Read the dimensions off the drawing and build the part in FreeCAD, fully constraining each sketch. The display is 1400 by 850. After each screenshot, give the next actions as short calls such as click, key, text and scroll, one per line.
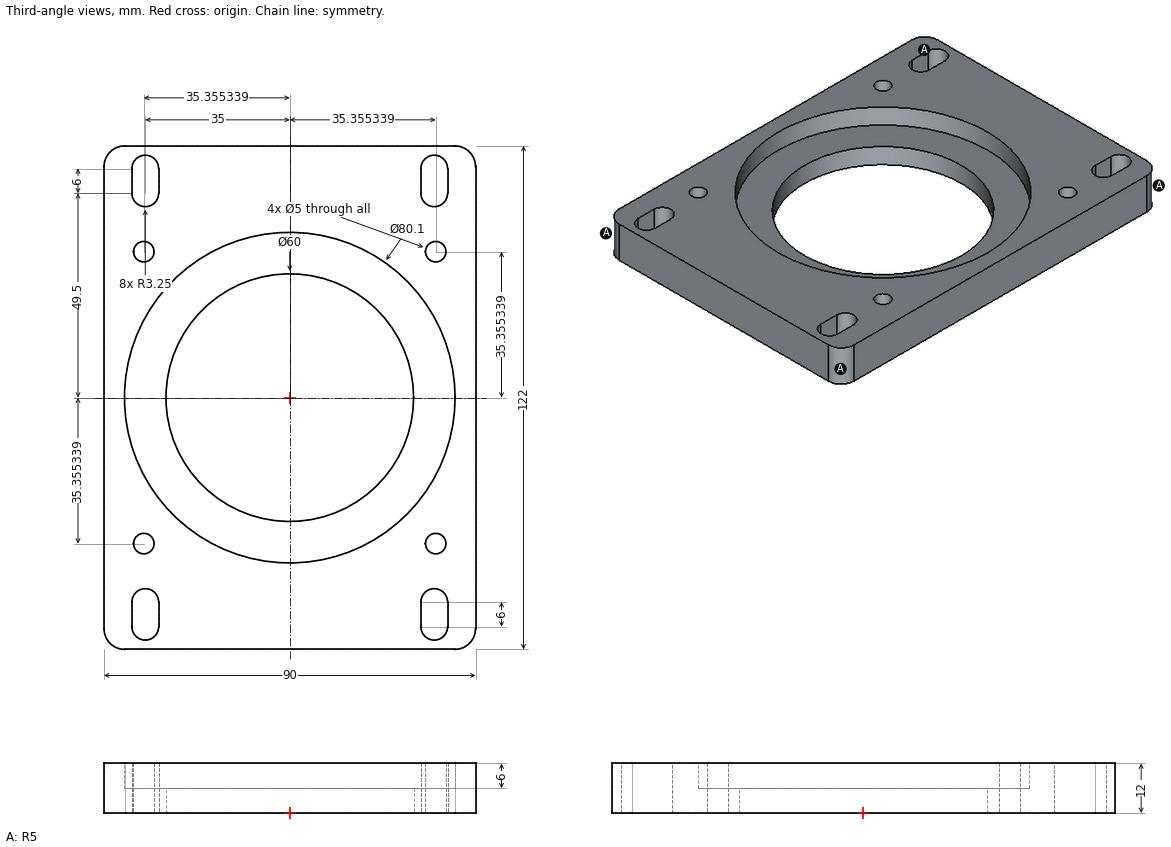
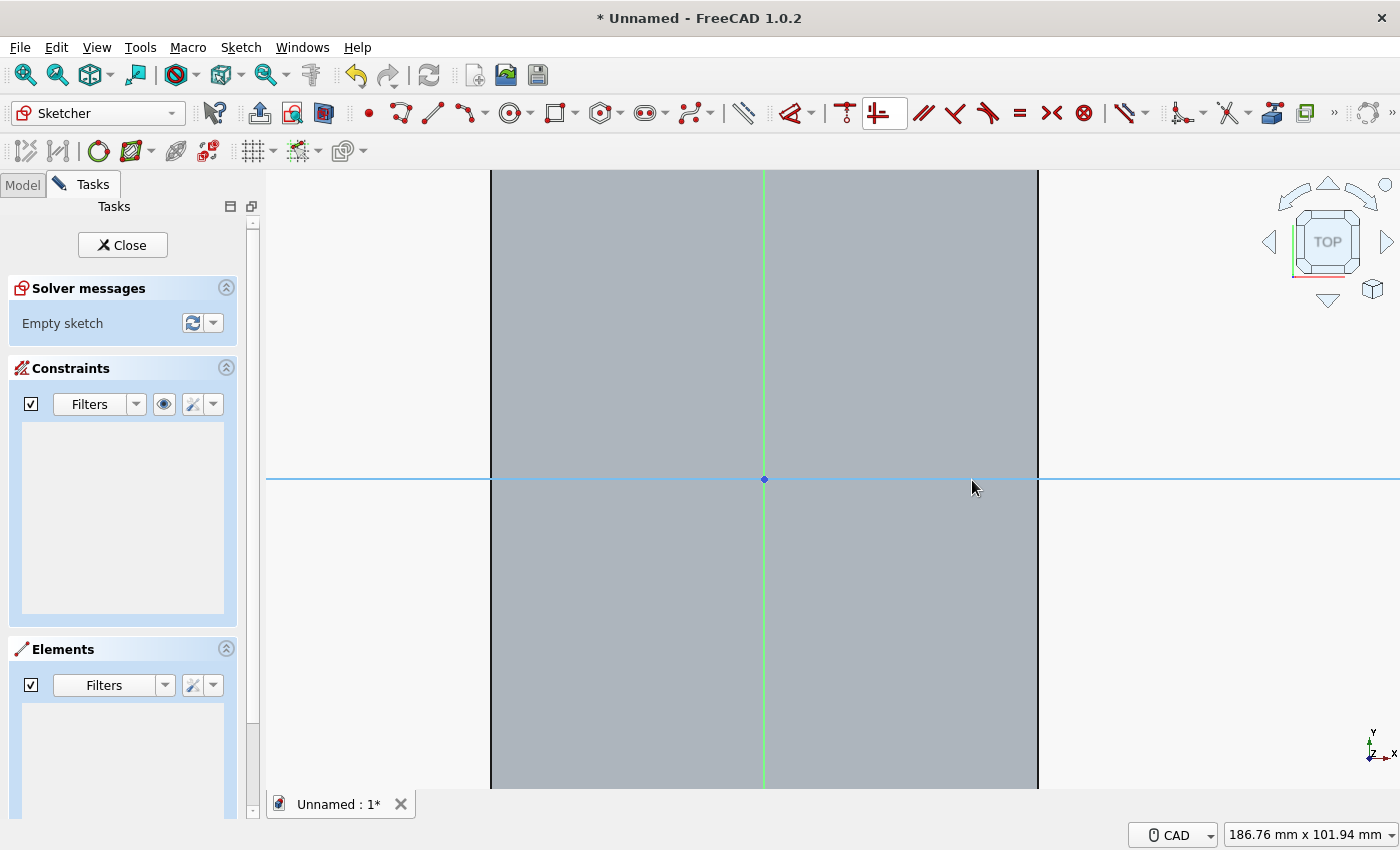
click(510, 114)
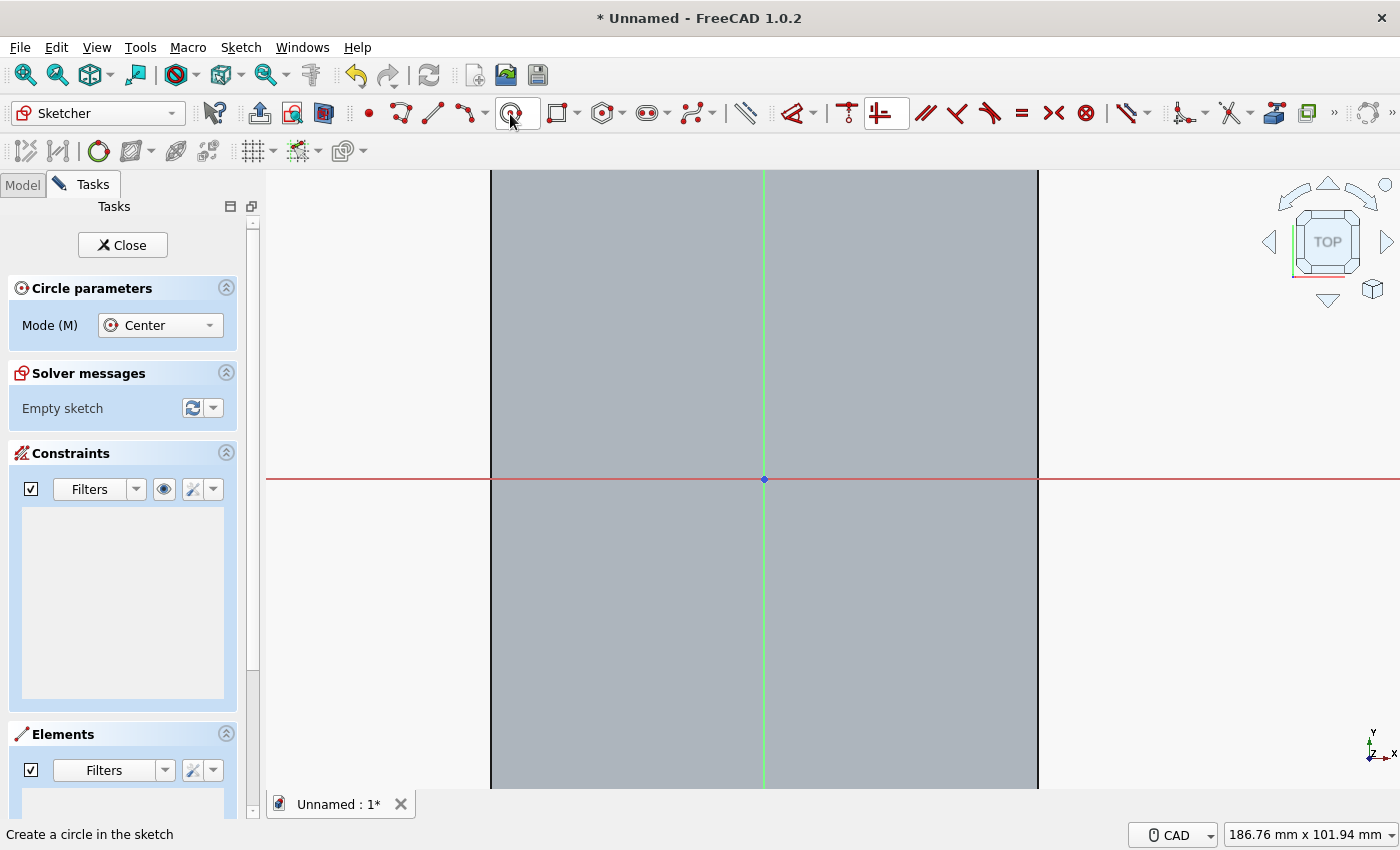
click(764, 479)
move(893, 350)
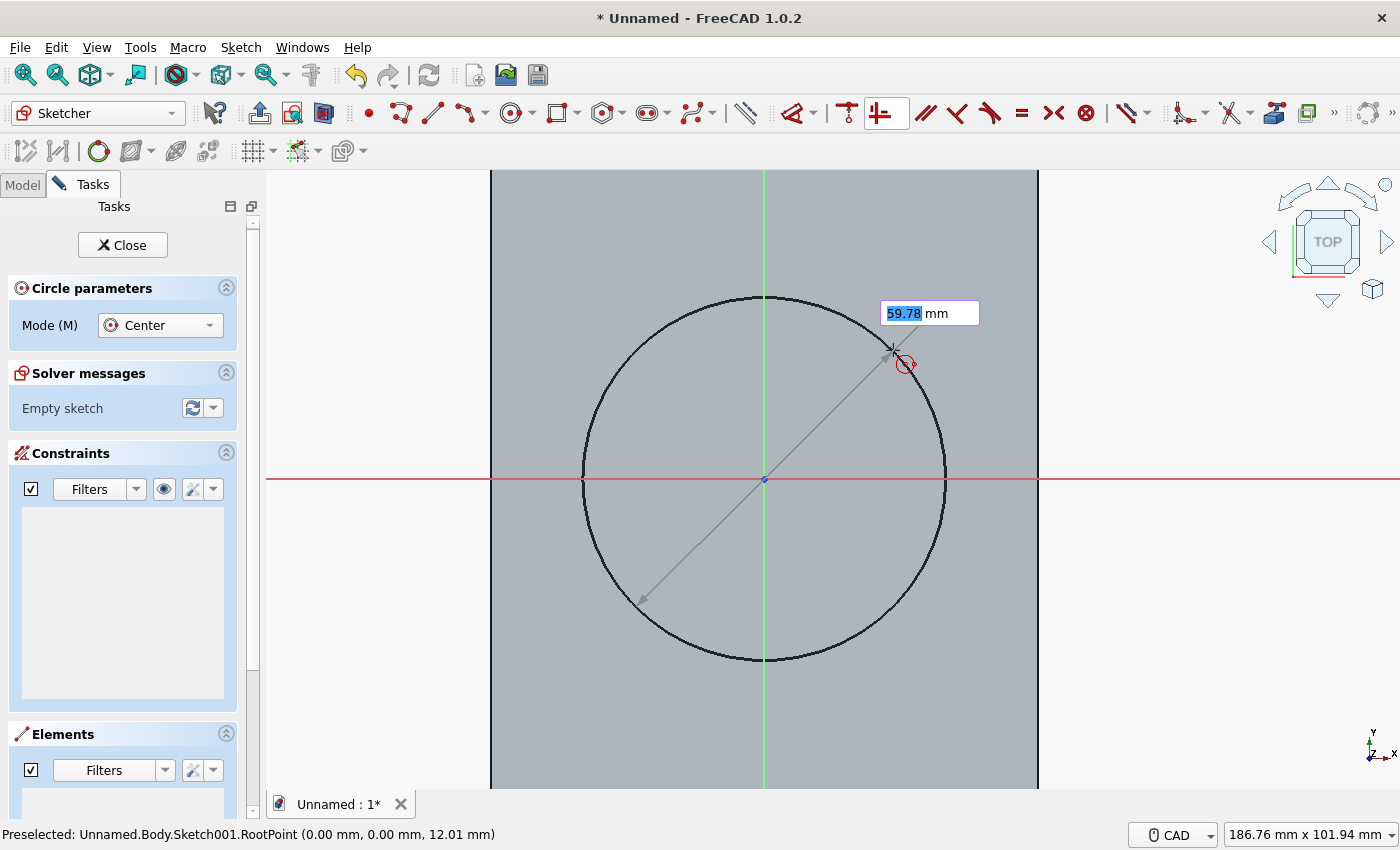
text(60)
key(Return)
key(Escape)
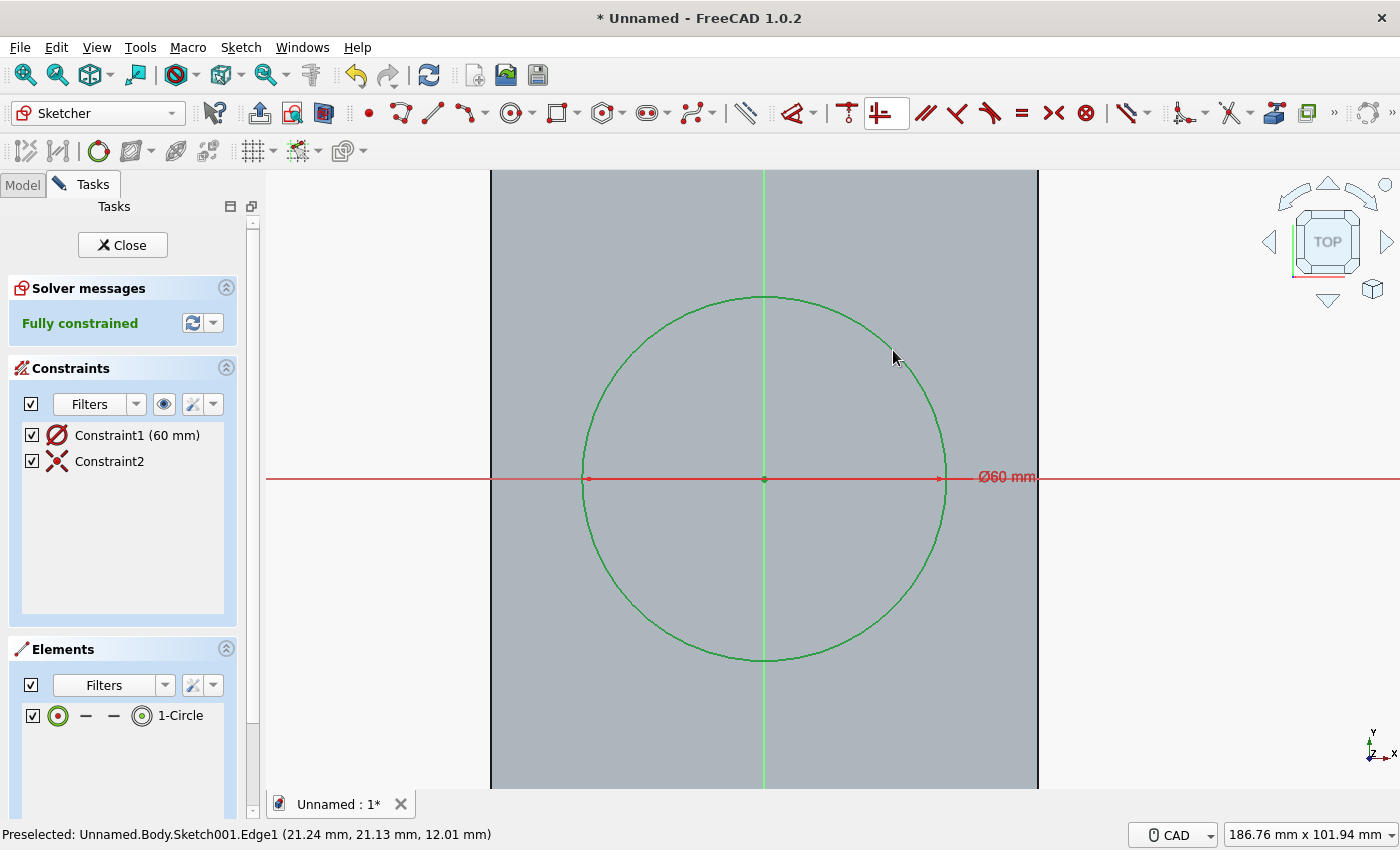
click(123, 245)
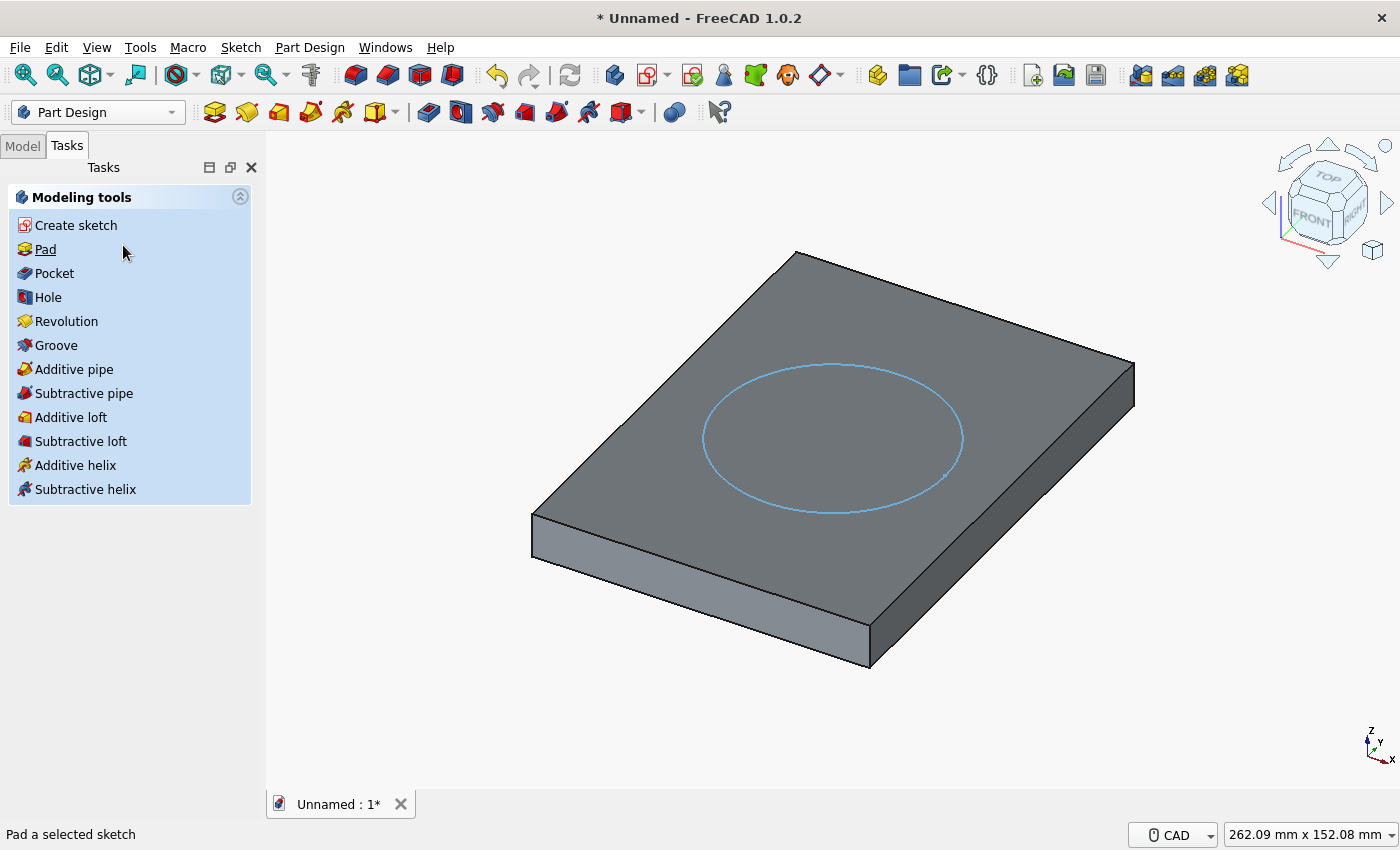
click(430, 112)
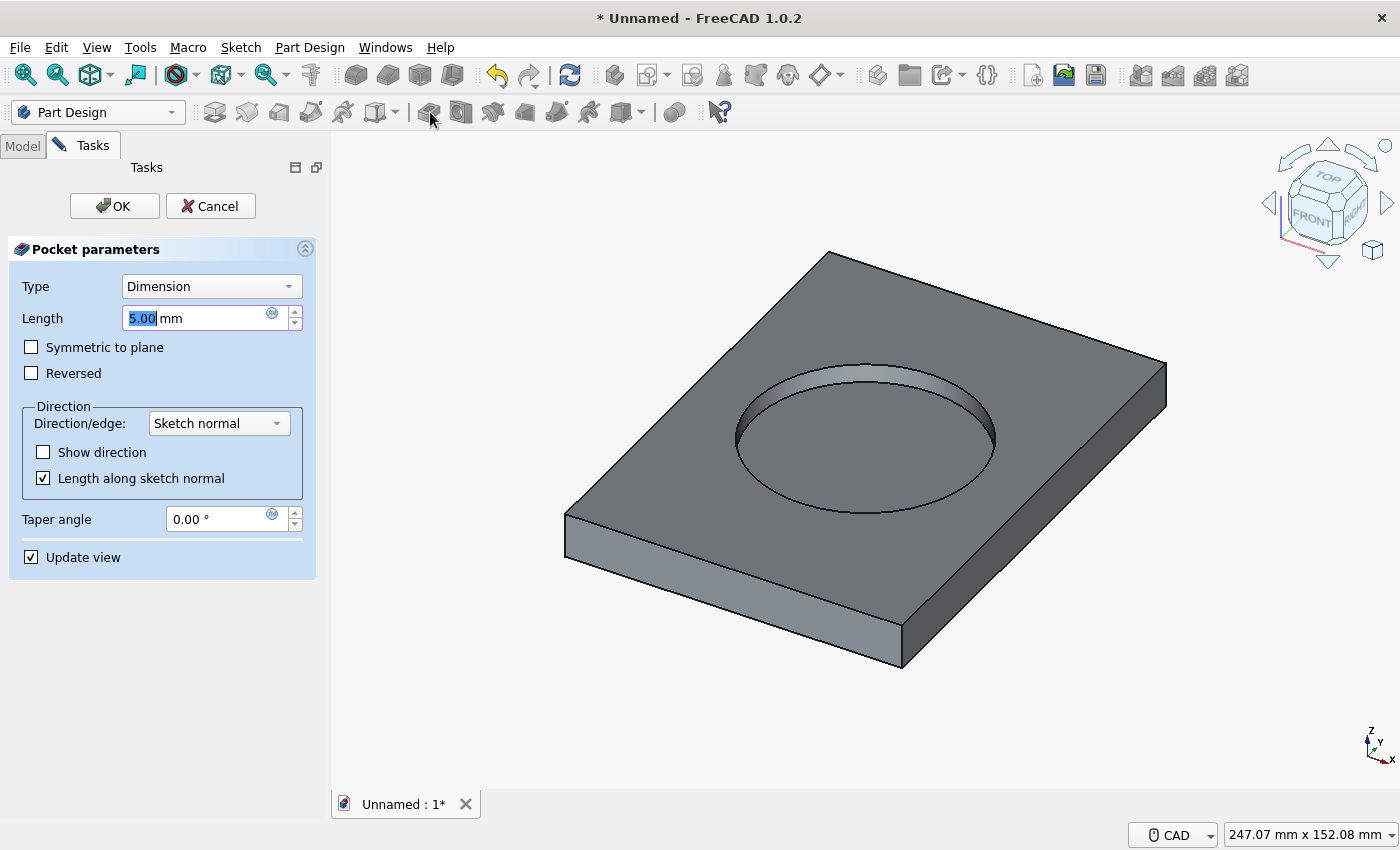
click(212, 286)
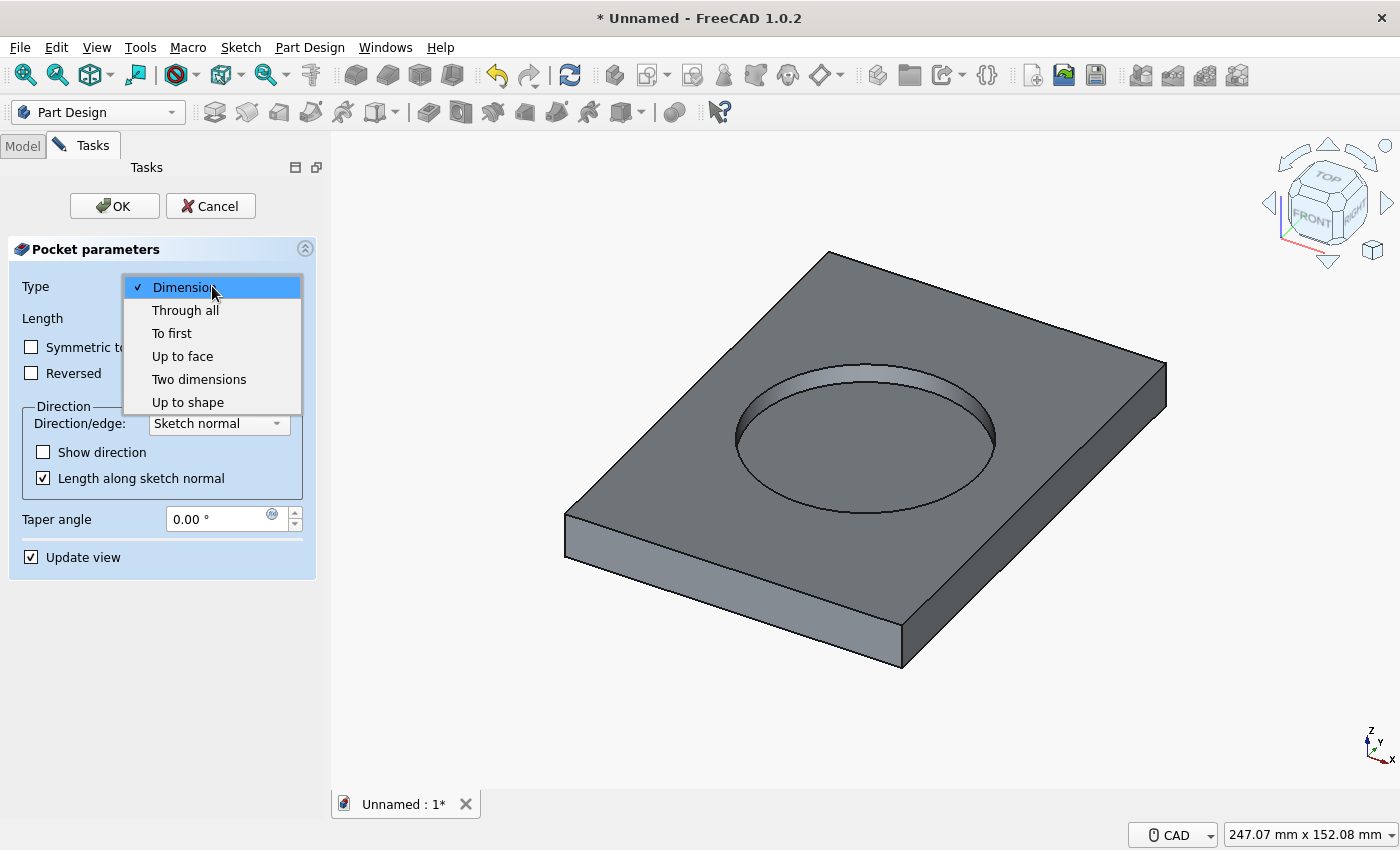
click(212, 310)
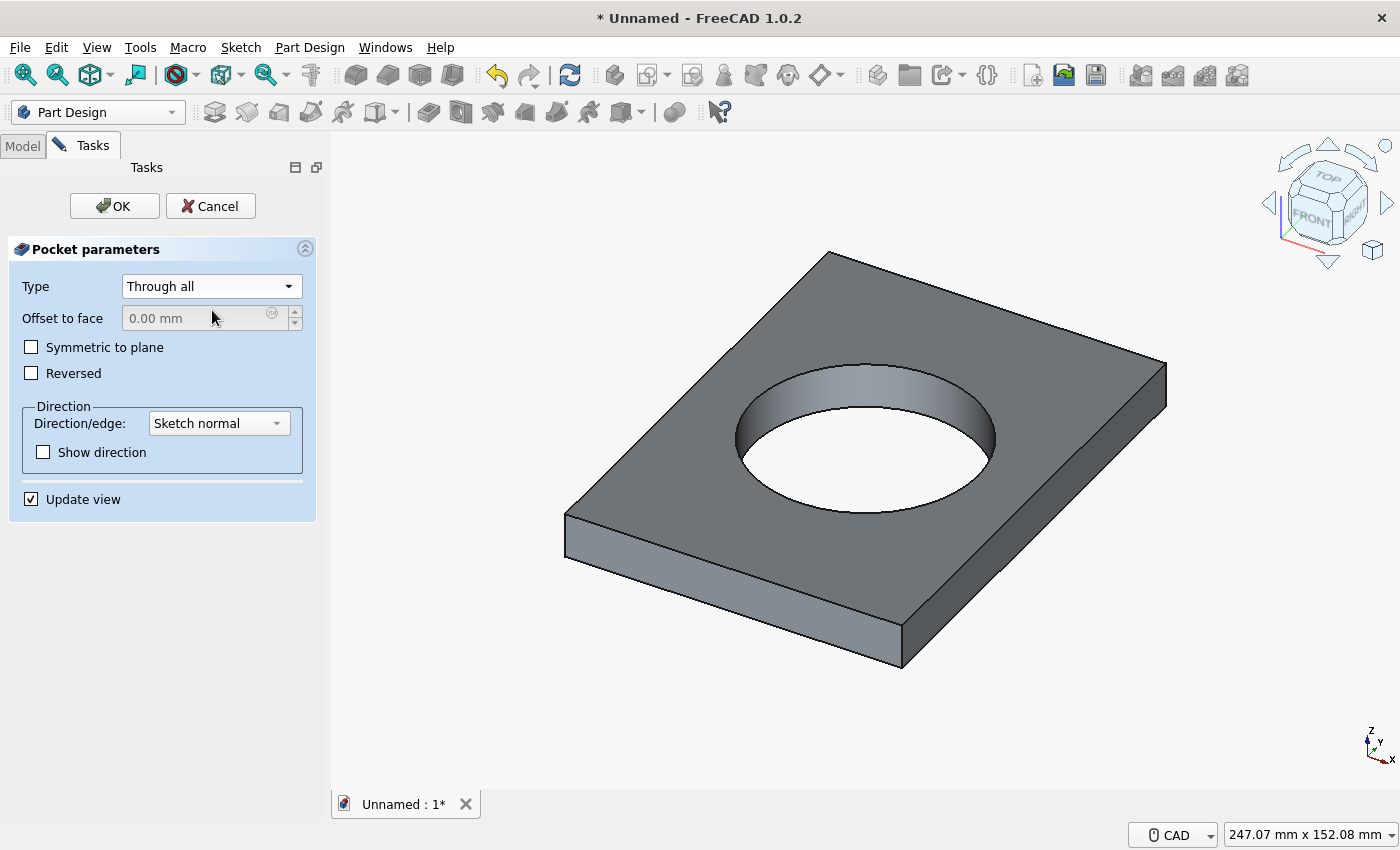
click(115, 206)